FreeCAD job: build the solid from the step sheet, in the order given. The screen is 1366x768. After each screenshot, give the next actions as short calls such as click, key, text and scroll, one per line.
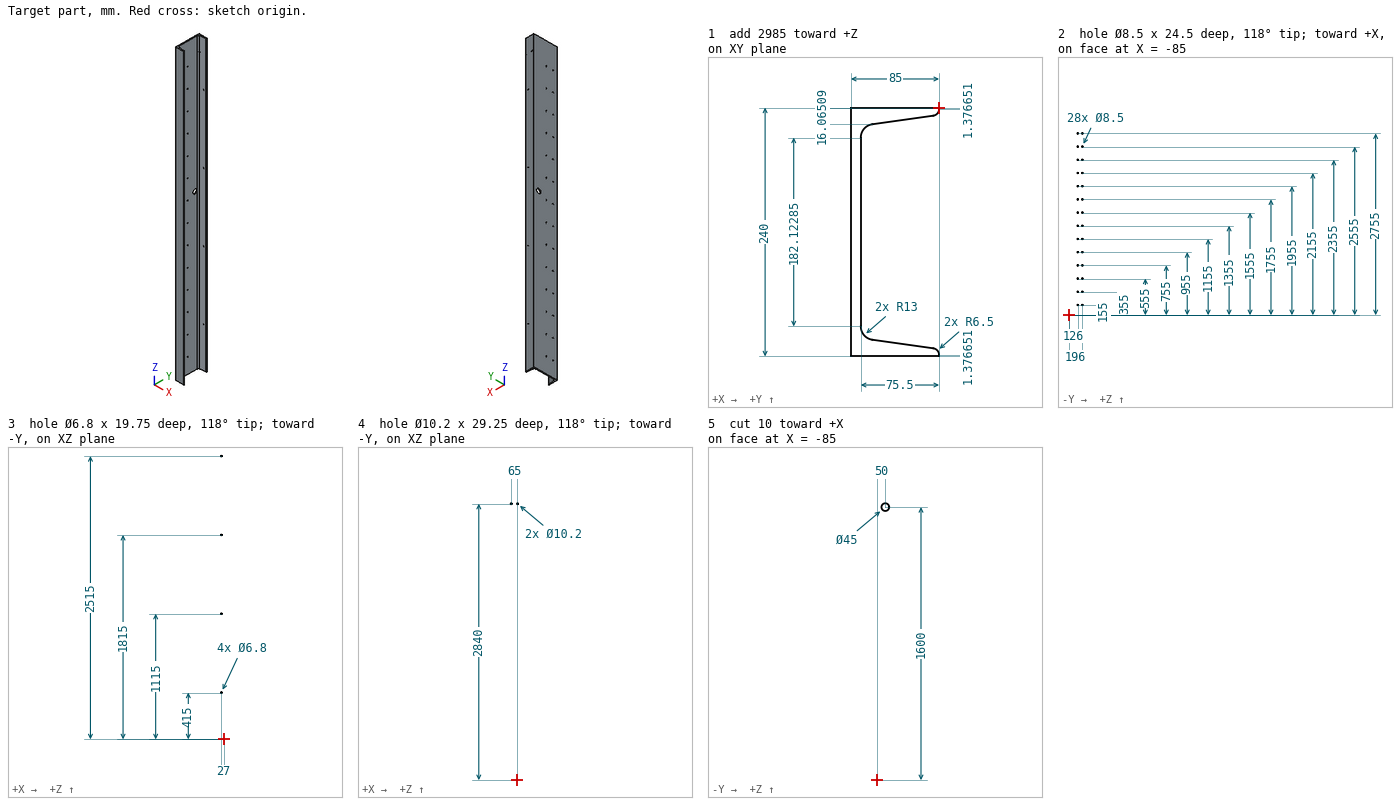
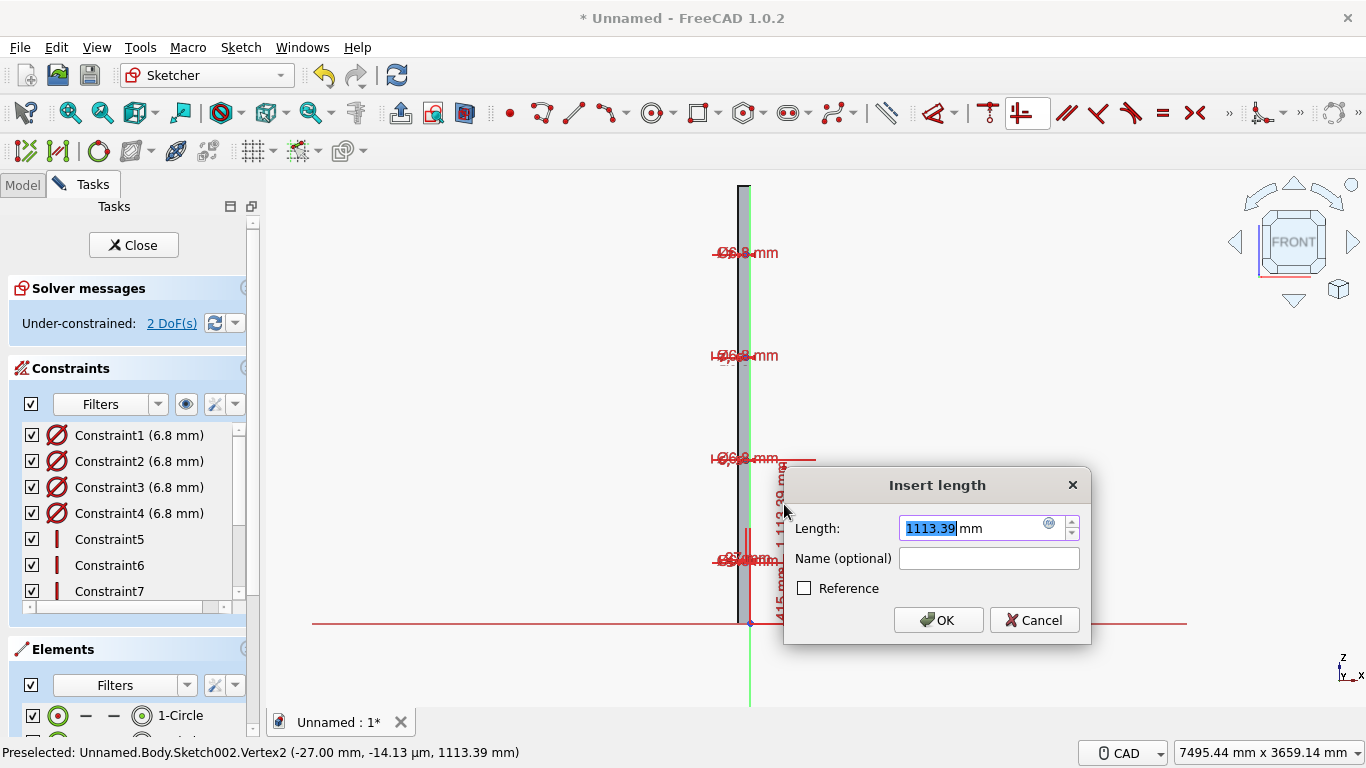
text(1115)
key(Return)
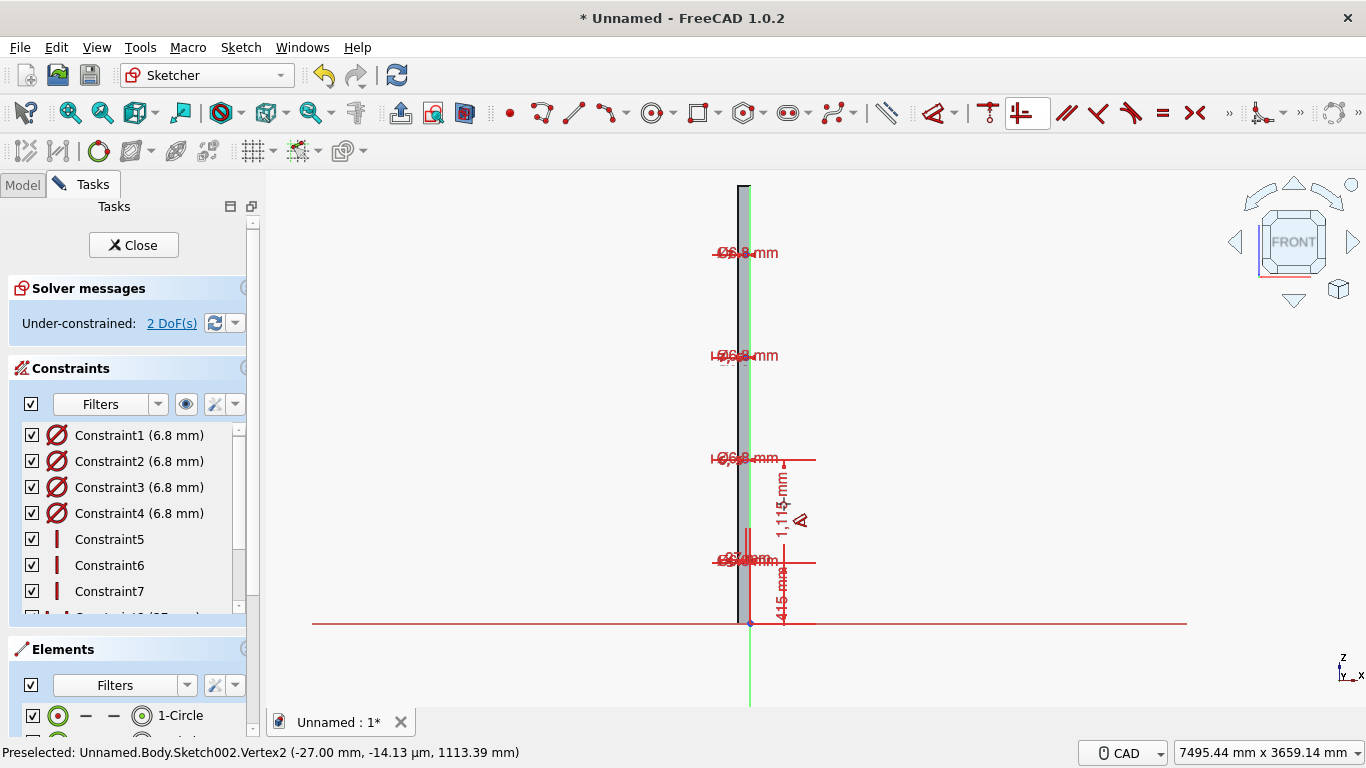
click(746, 358)
click(784, 429)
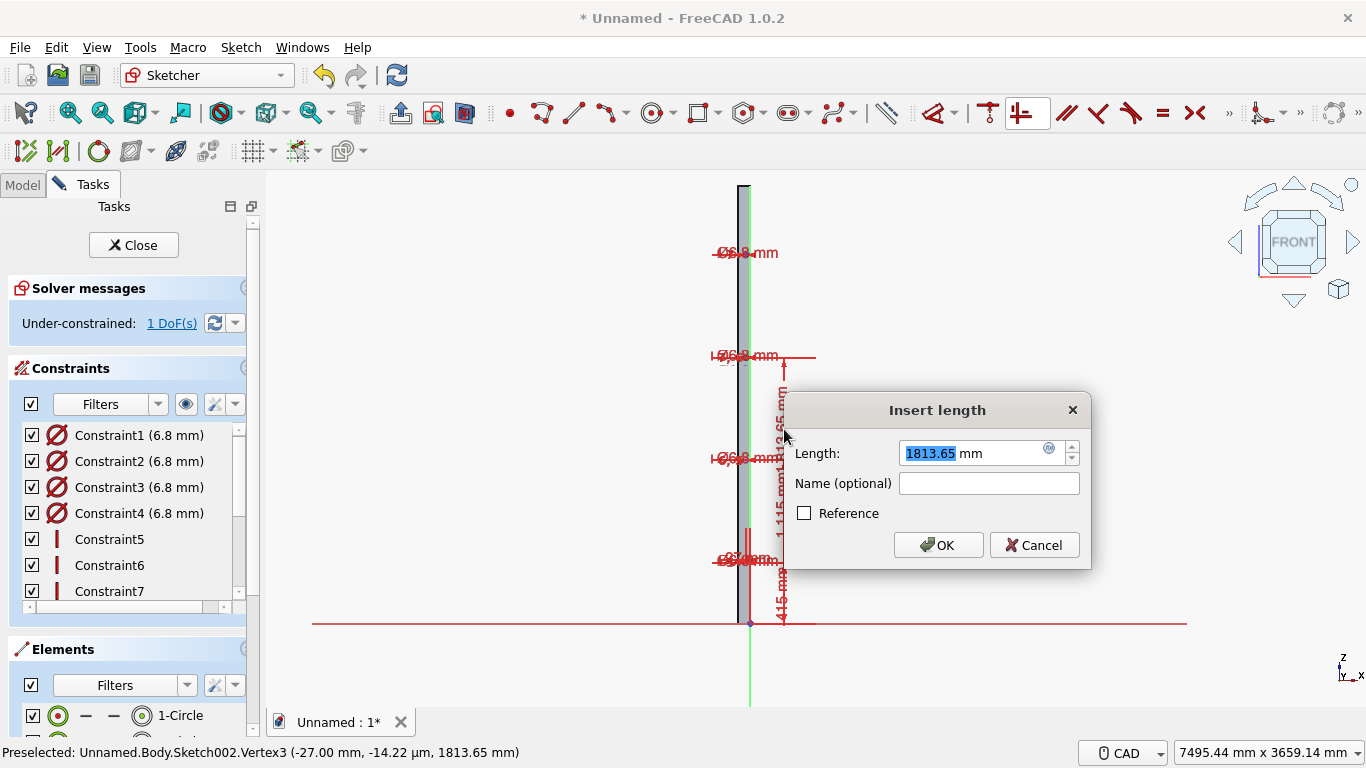
text(1815)
key(Return)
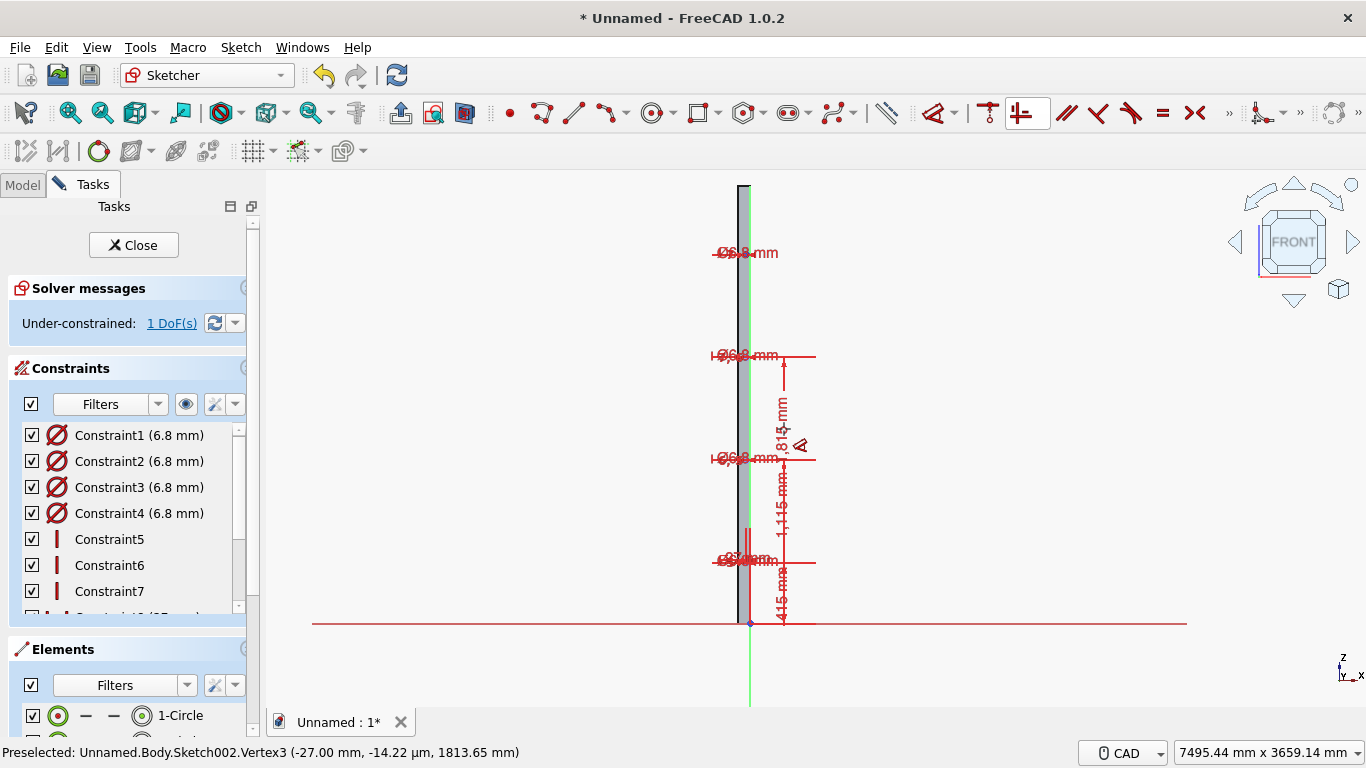
click(746, 255)
click(784, 355)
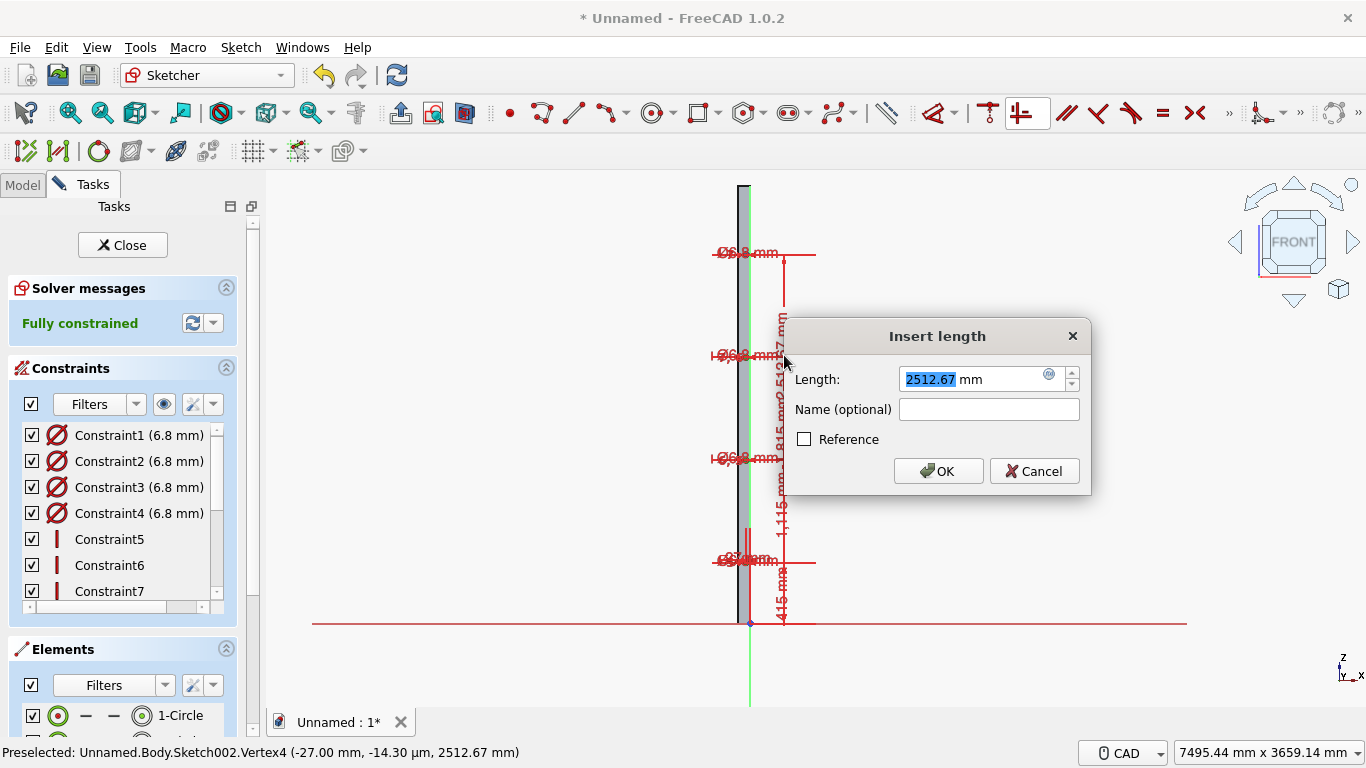
text(2515)
key(Return)
key(Escape)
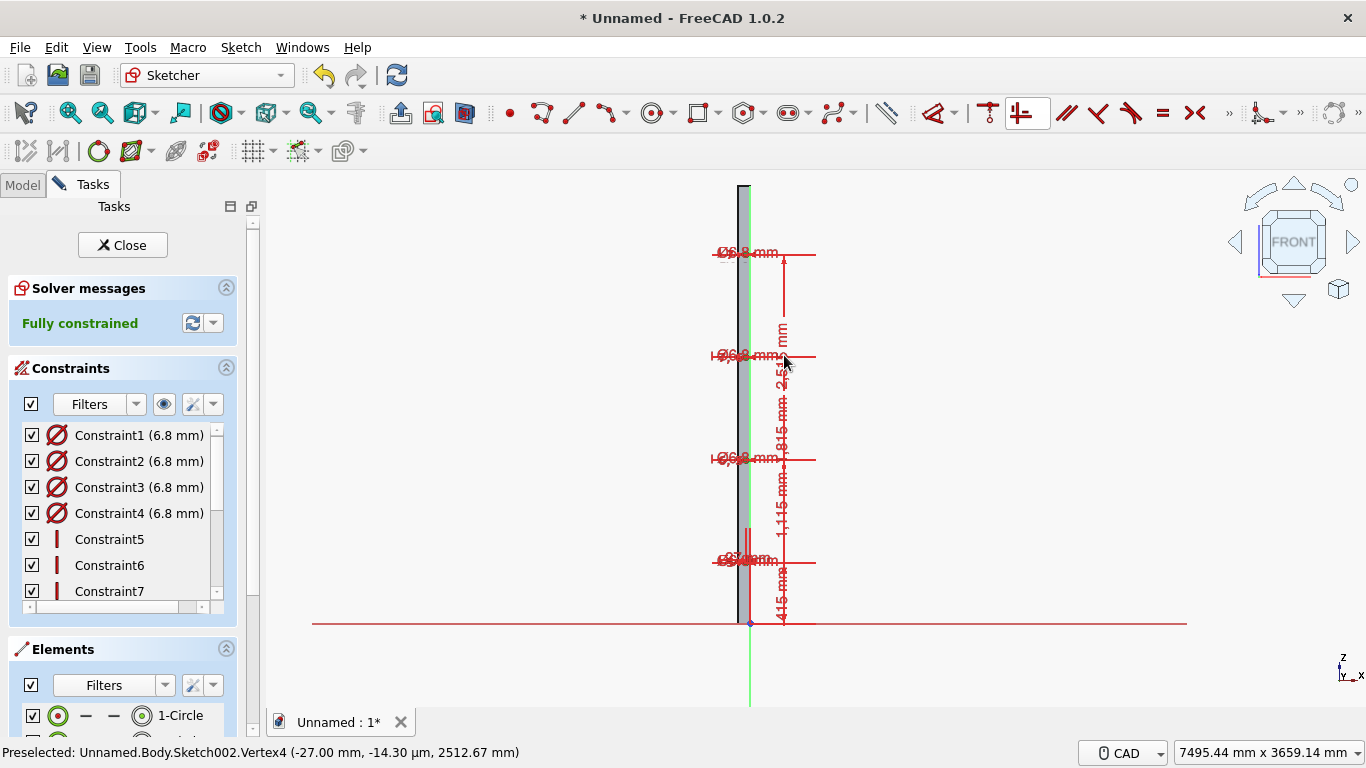
click(123, 245)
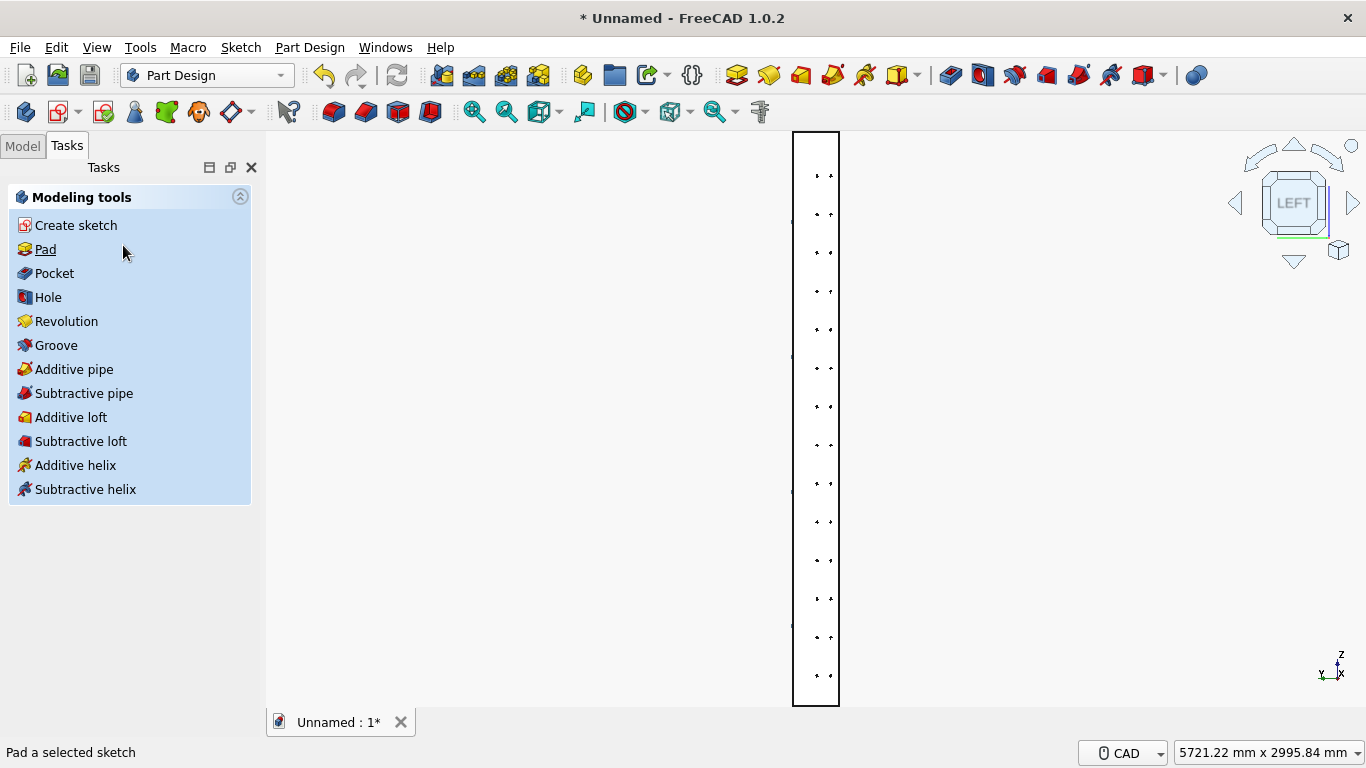
click(984, 76)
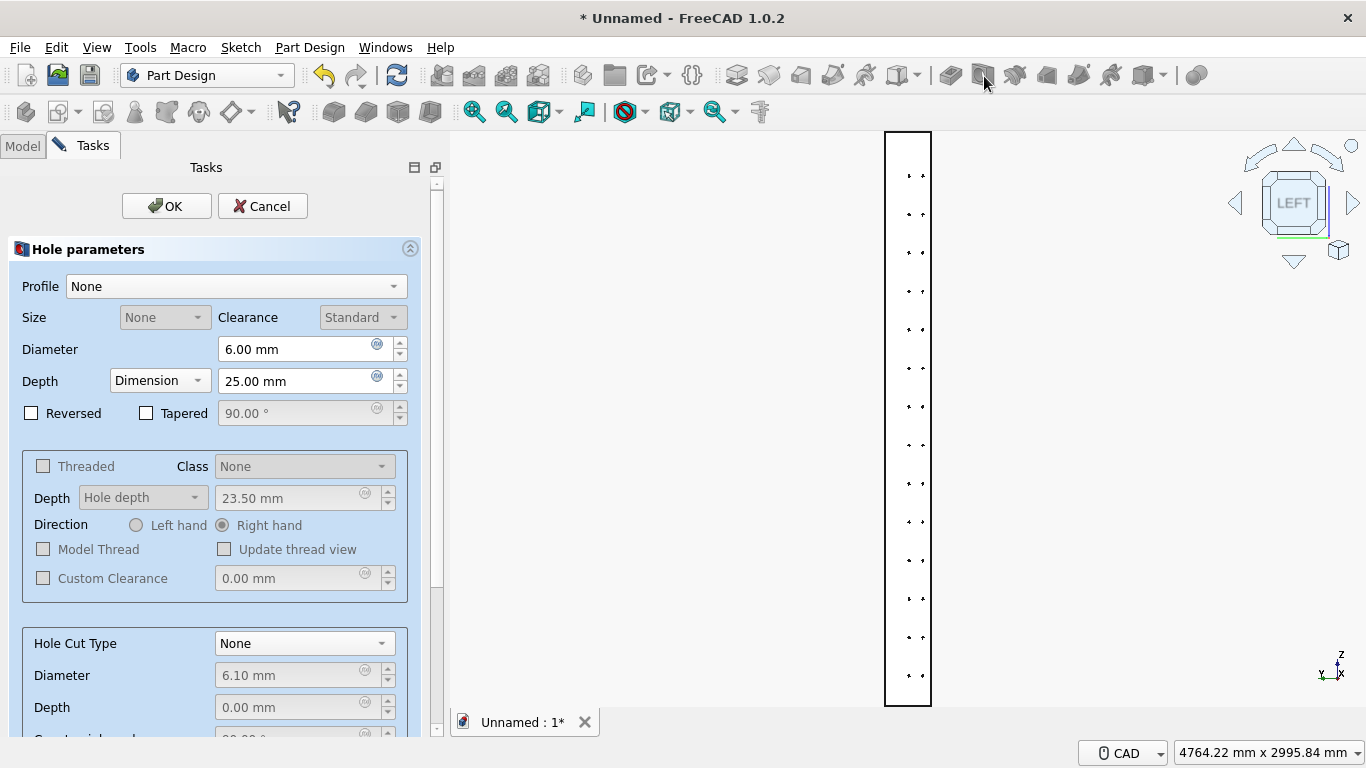
triple_click(305, 349)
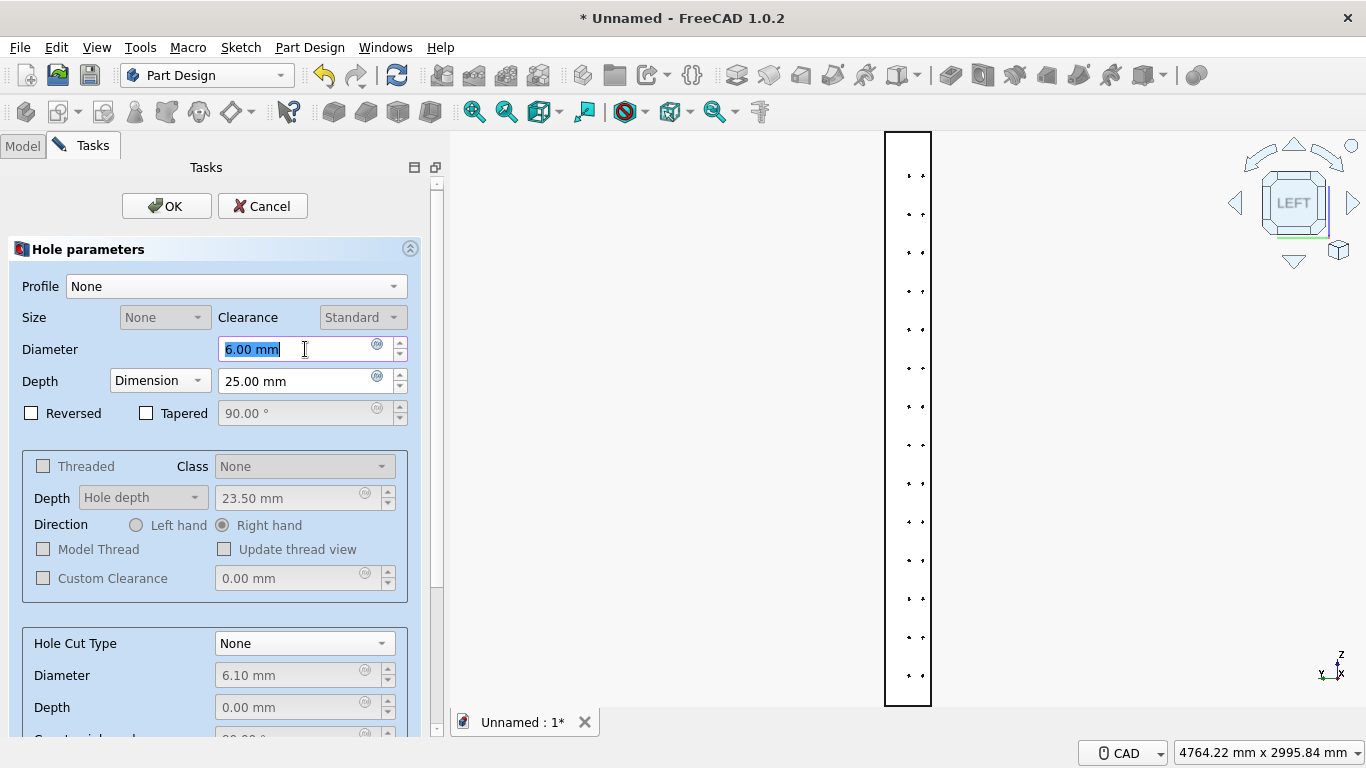
text(6.8)
key(Tab)